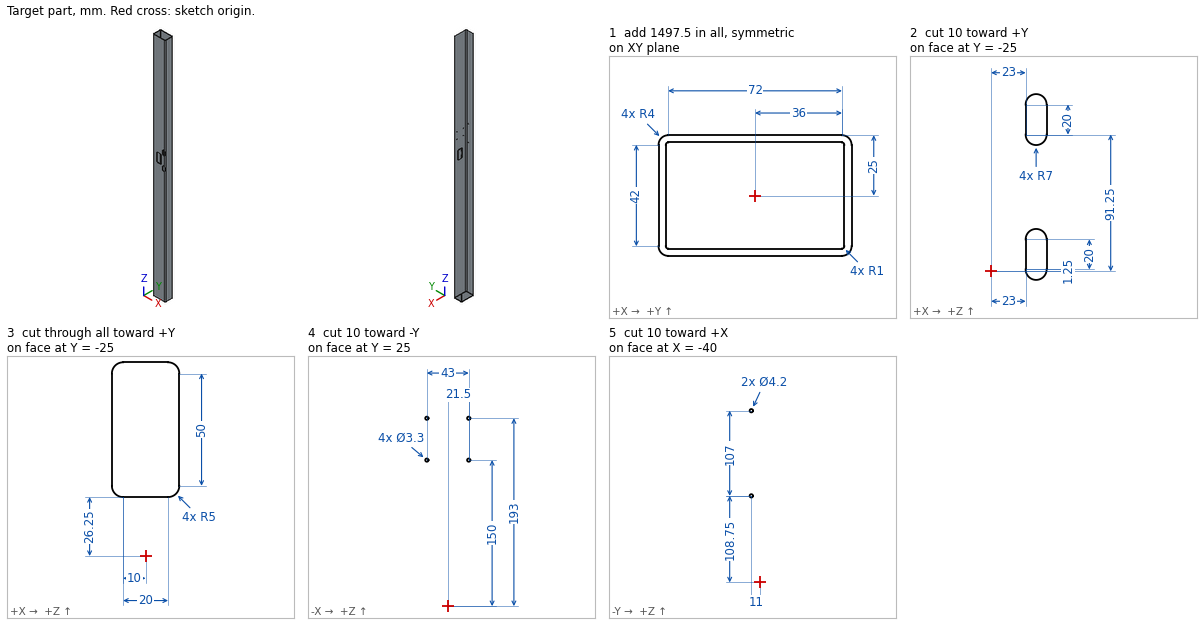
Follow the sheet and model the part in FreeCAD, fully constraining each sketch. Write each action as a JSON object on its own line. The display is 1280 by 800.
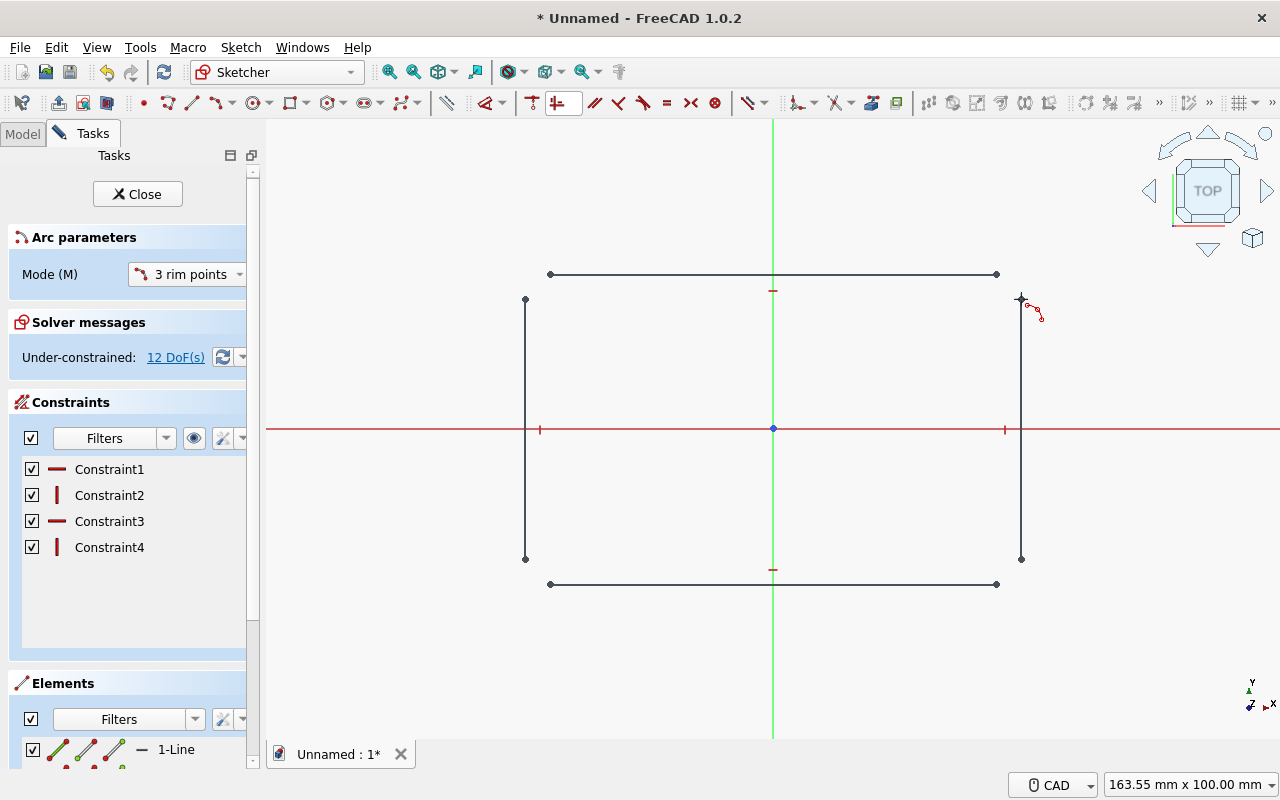
{"action": "left_click", "coordinate": [550, 275]}
{"action": "left_click", "coordinate": [525, 300]}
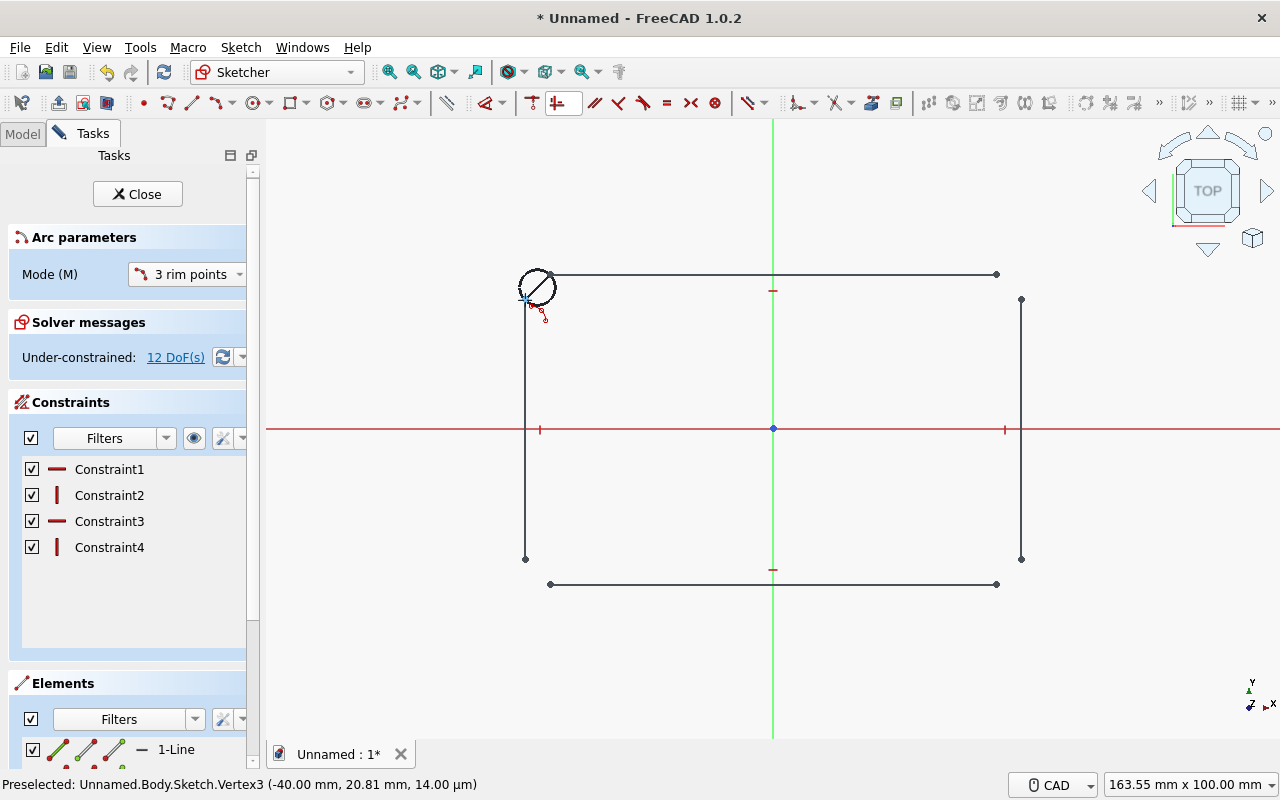
{"action": "scroll", "coordinate": [532, 281], "scroll_direction": "up", "scroll_amount": 4}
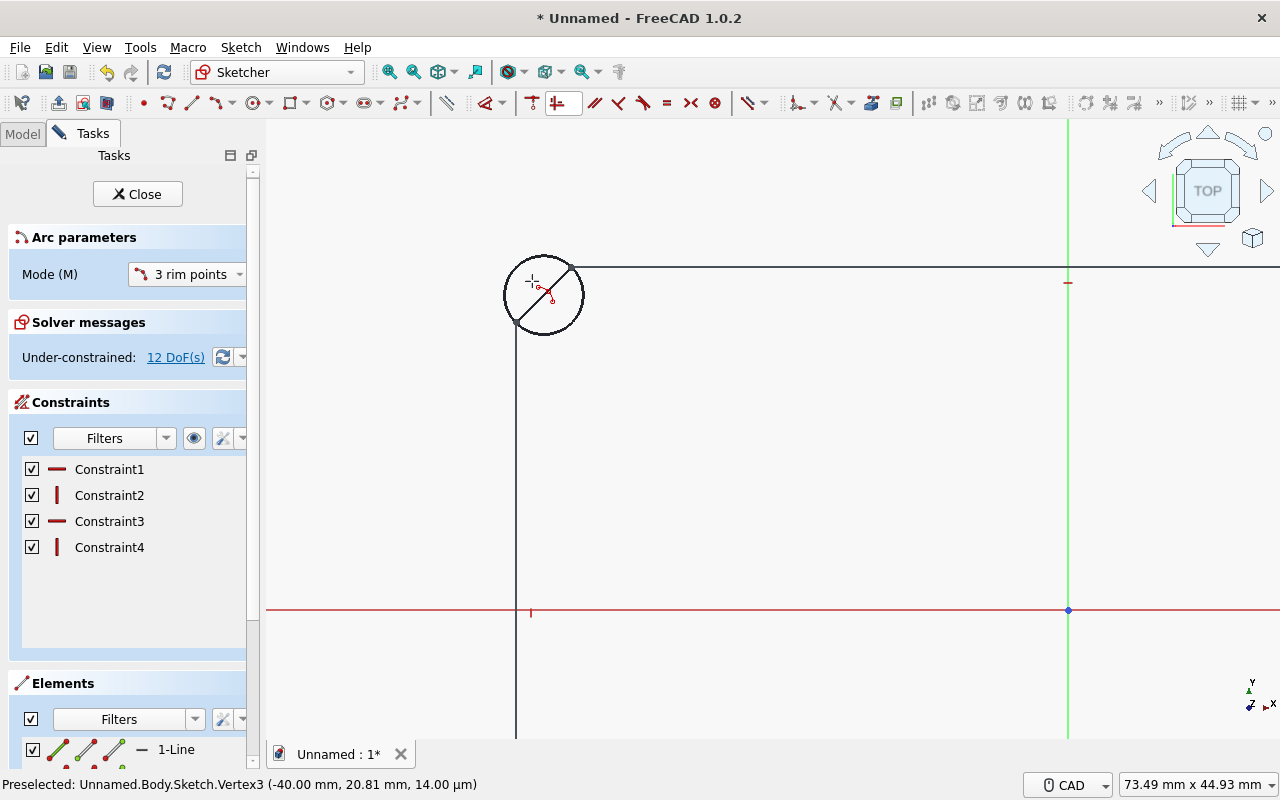
{"action": "left_click", "coordinate": [532, 281]}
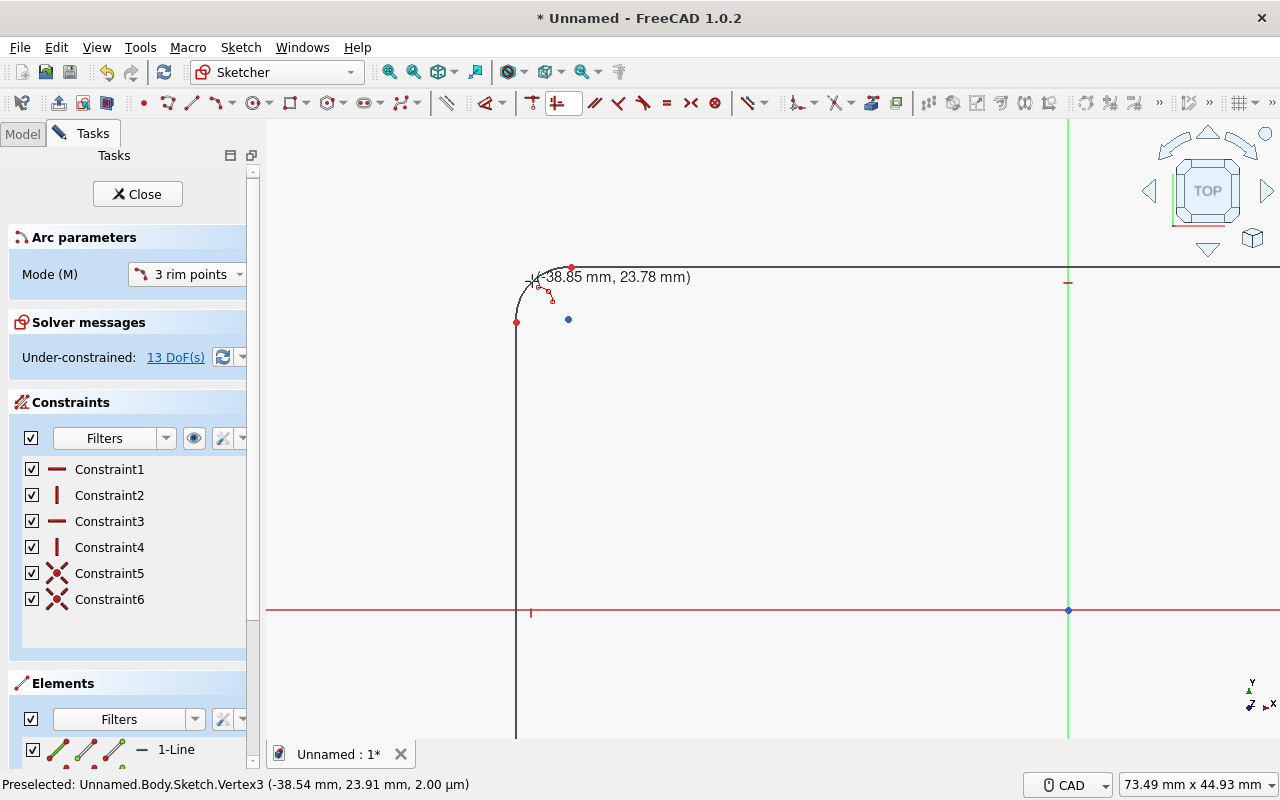
{"action": "scroll", "coordinate": [294, 209], "scroll_direction": "down", "scroll_amount": 3}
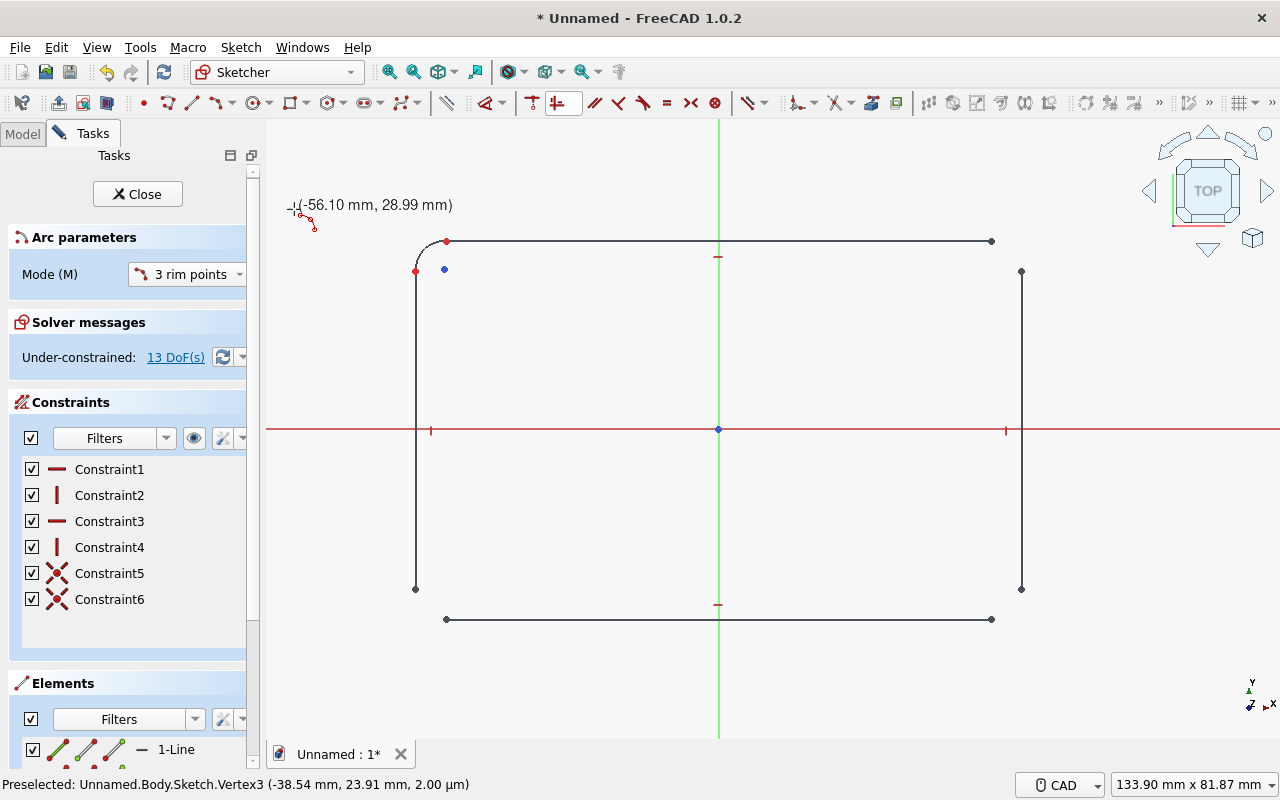
{"action": "left_click", "coordinate": [416, 589]}
{"action": "left_click", "coordinate": [446, 620]}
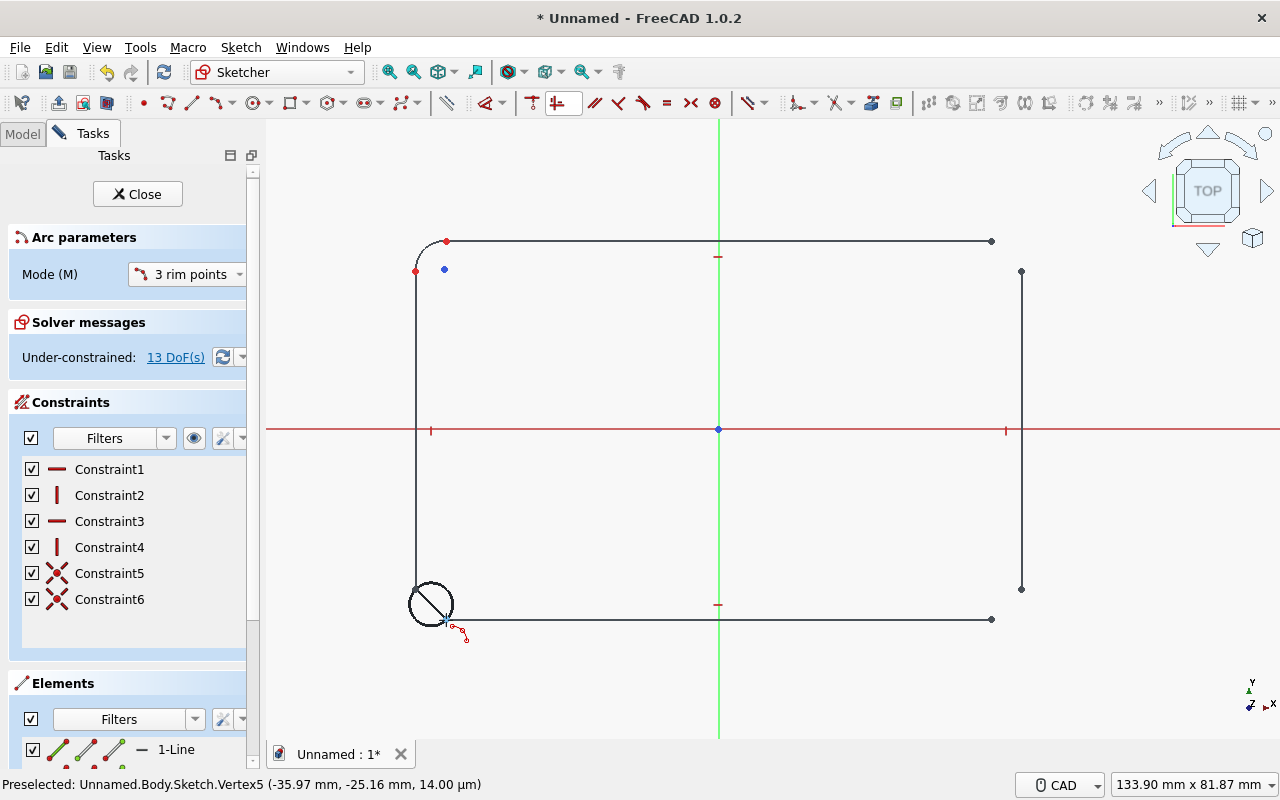
{"action": "scroll", "coordinate": [425, 610], "scroll_direction": "up", "scroll_amount": 3}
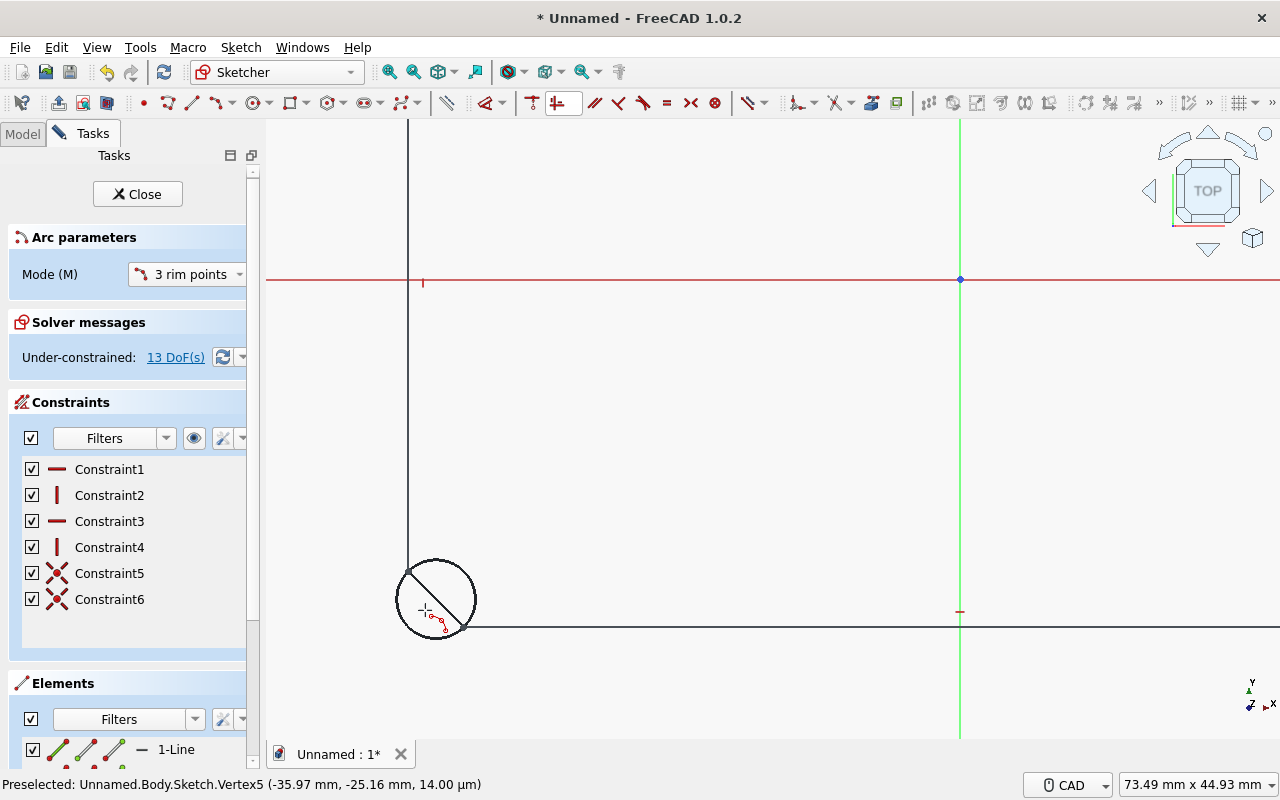
{"action": "left_click", "coordinate": [424, 609]}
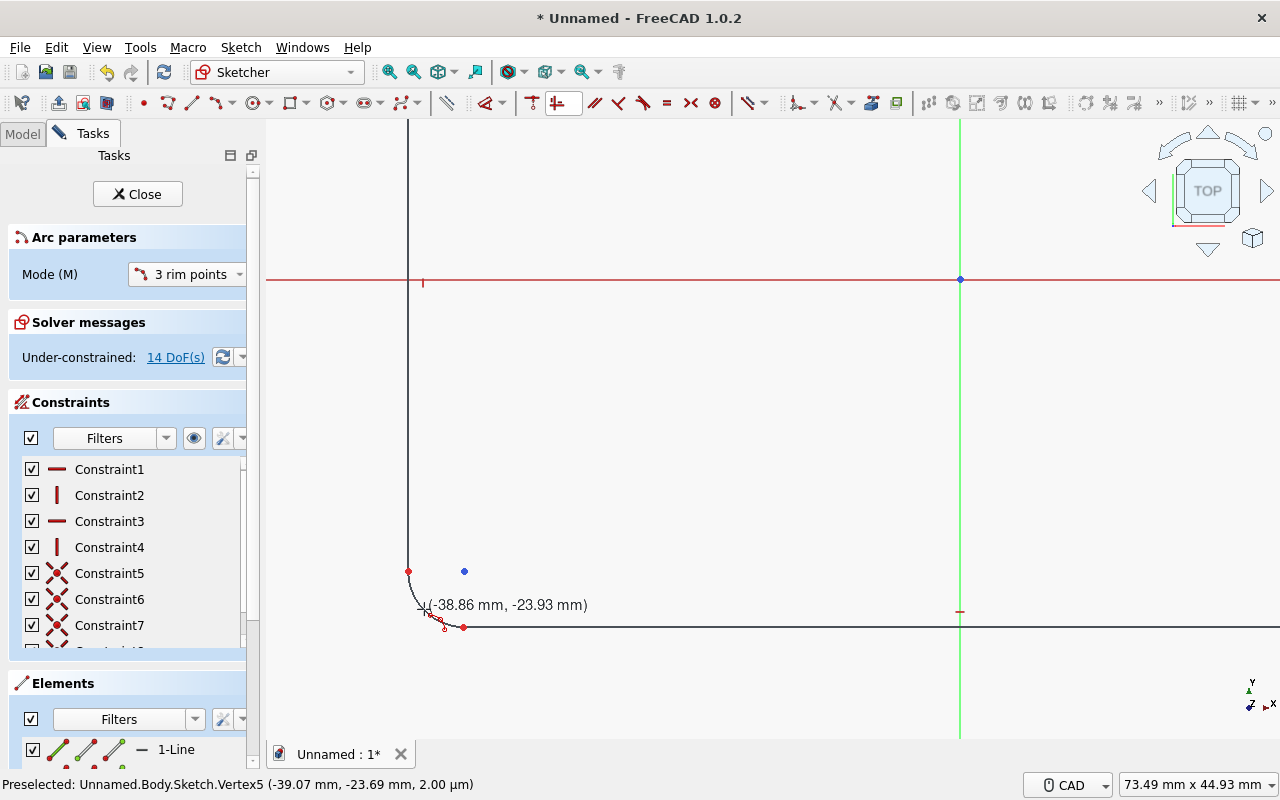
{"action": "scroll", "coordinate": [393, 610], "scroll_direction": "down", "scroll_amount": 3}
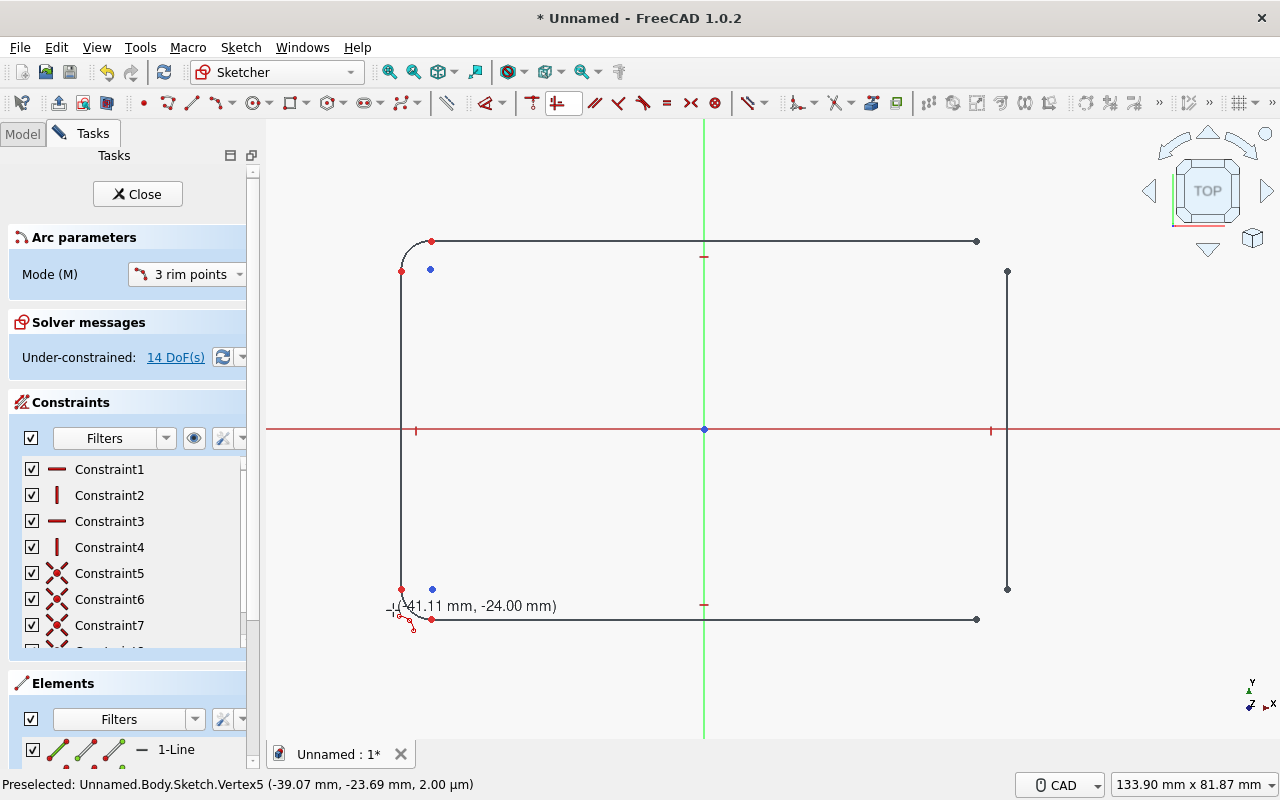
{"action": "left_click", "coordinate": [977, 620]}
{"action": "left_click", "coordinate": [1007, 589]}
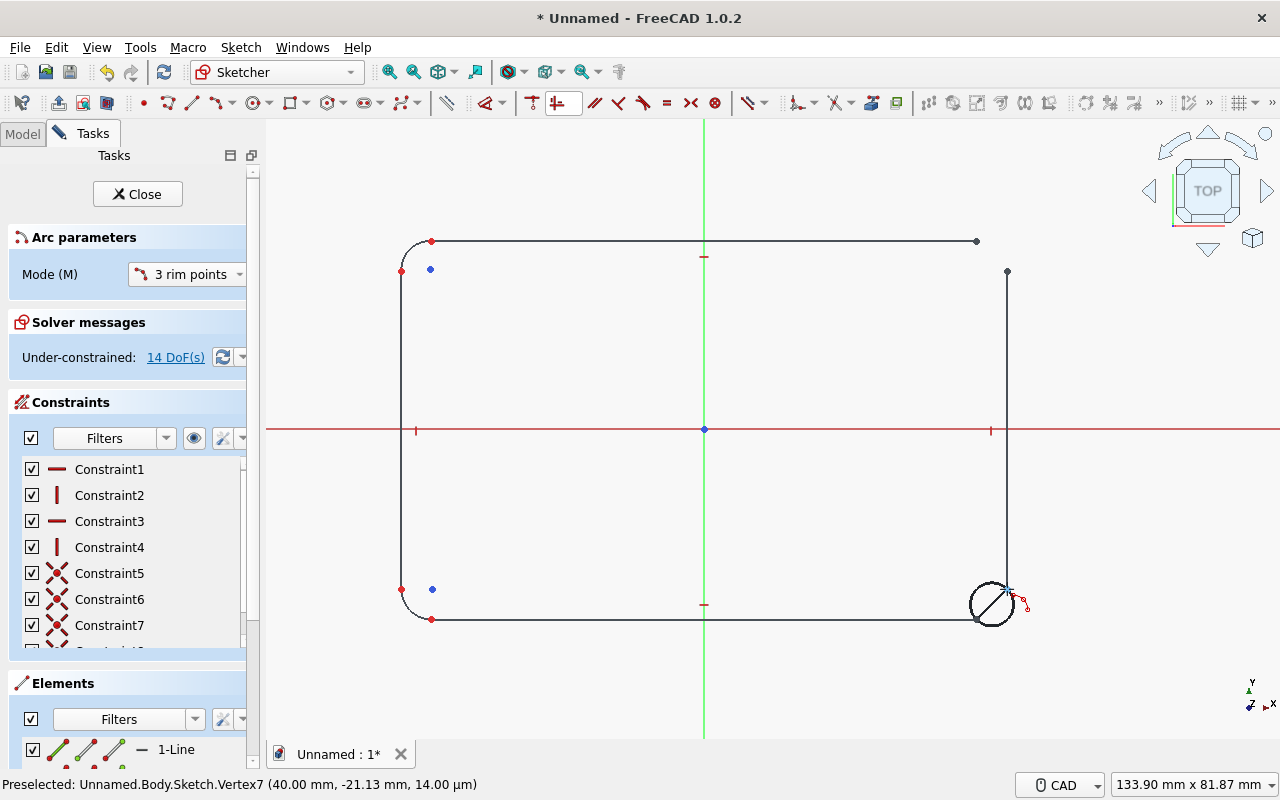
{"action": "scroll", "coordinate": [998, 610], "scroll_direction": "up", "scroll_amount": 3}